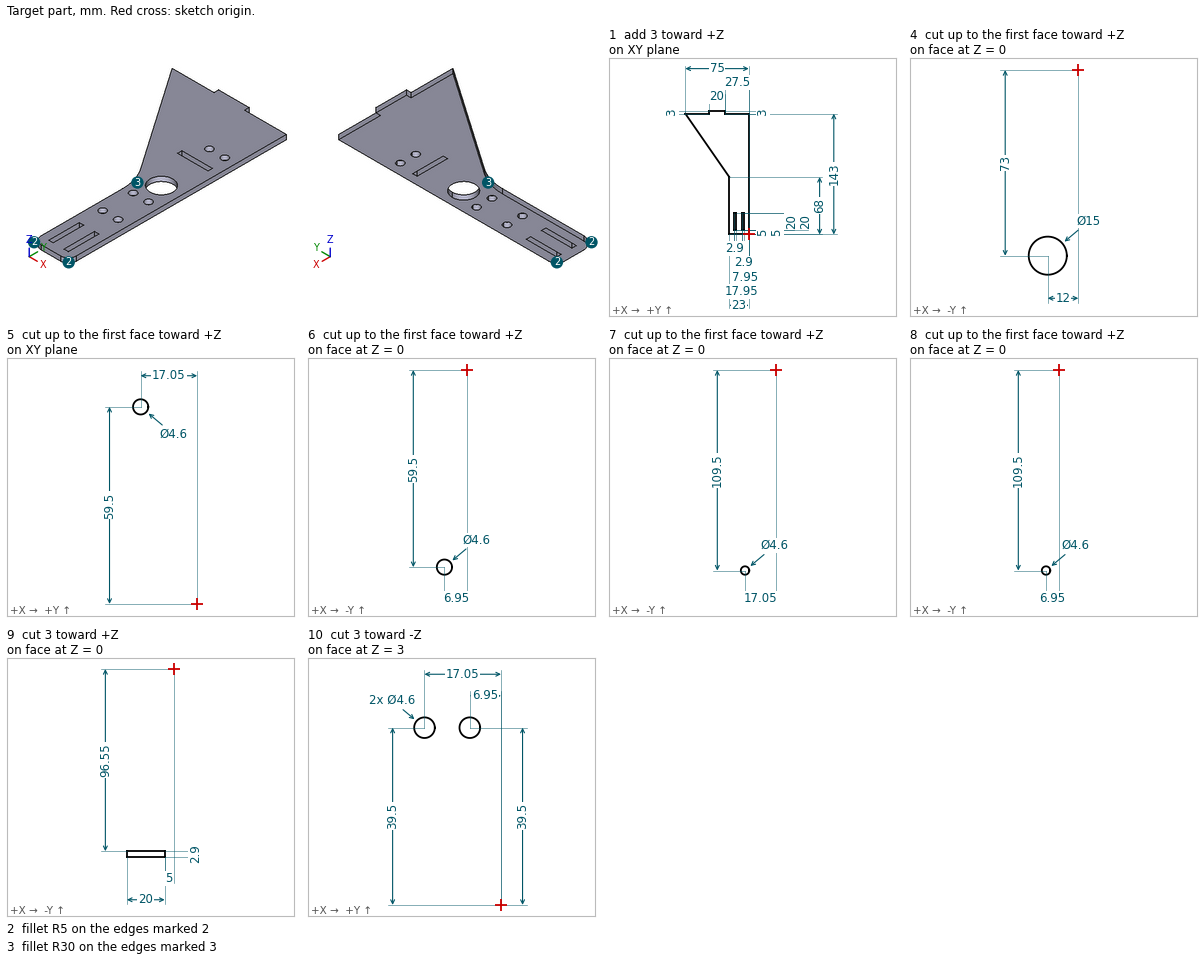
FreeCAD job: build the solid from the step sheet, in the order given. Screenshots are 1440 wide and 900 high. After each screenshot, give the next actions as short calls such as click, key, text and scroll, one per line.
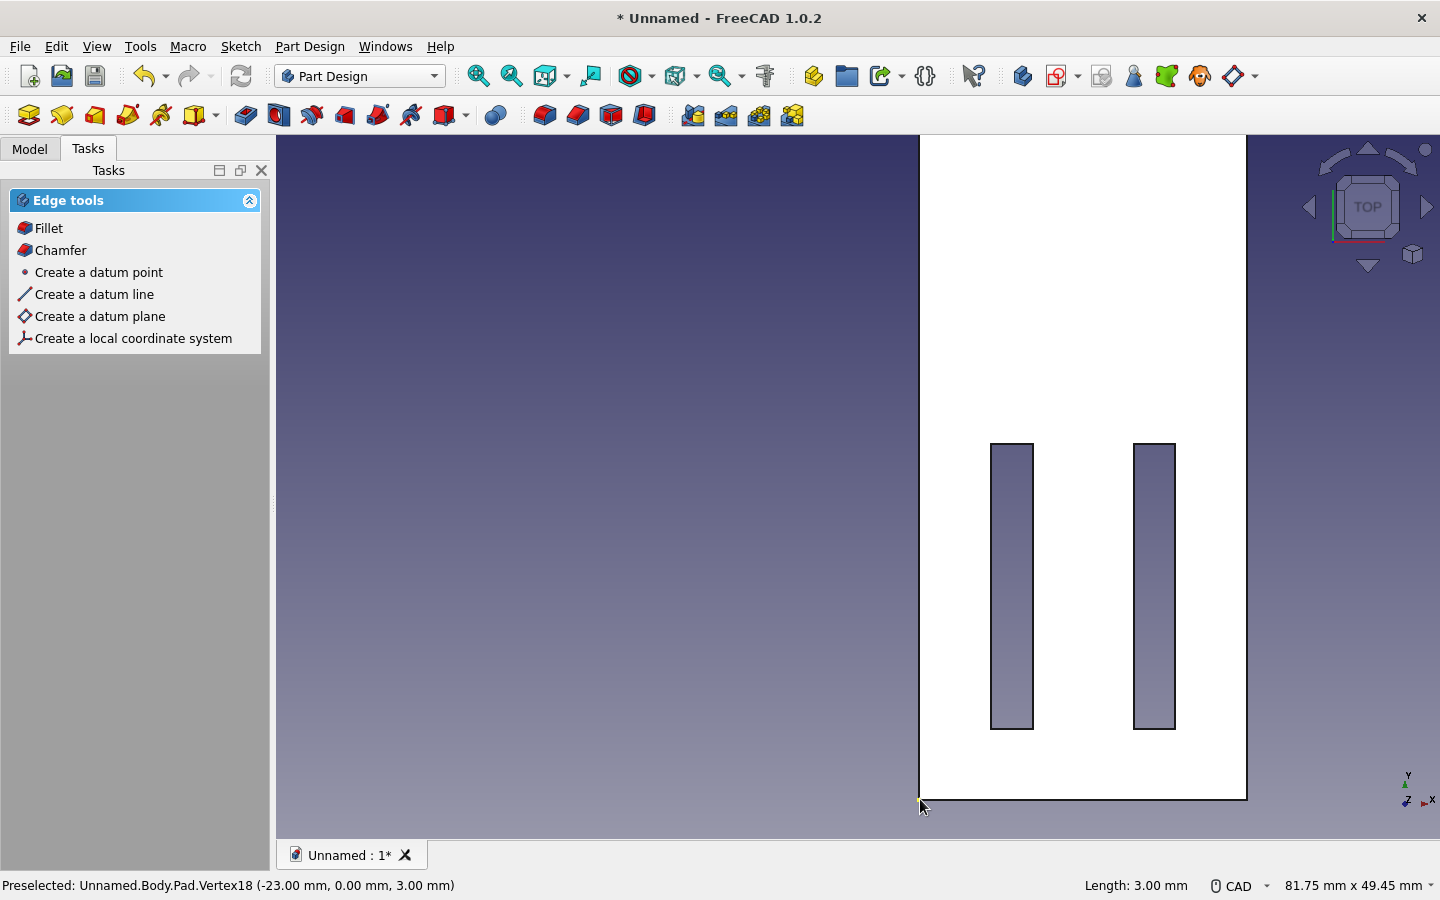
key(v)
key(f)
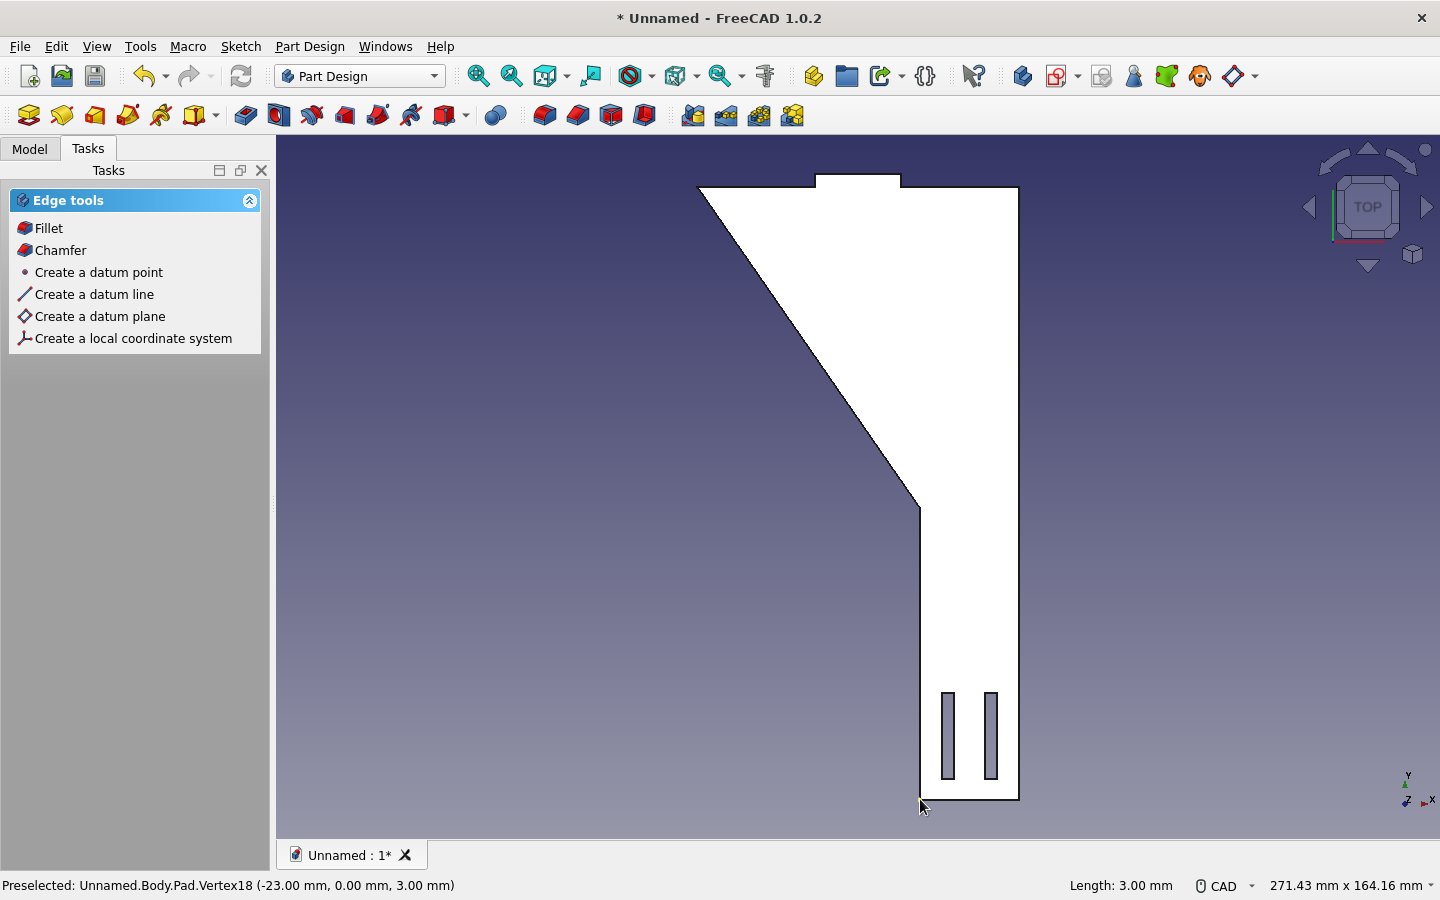
key(1)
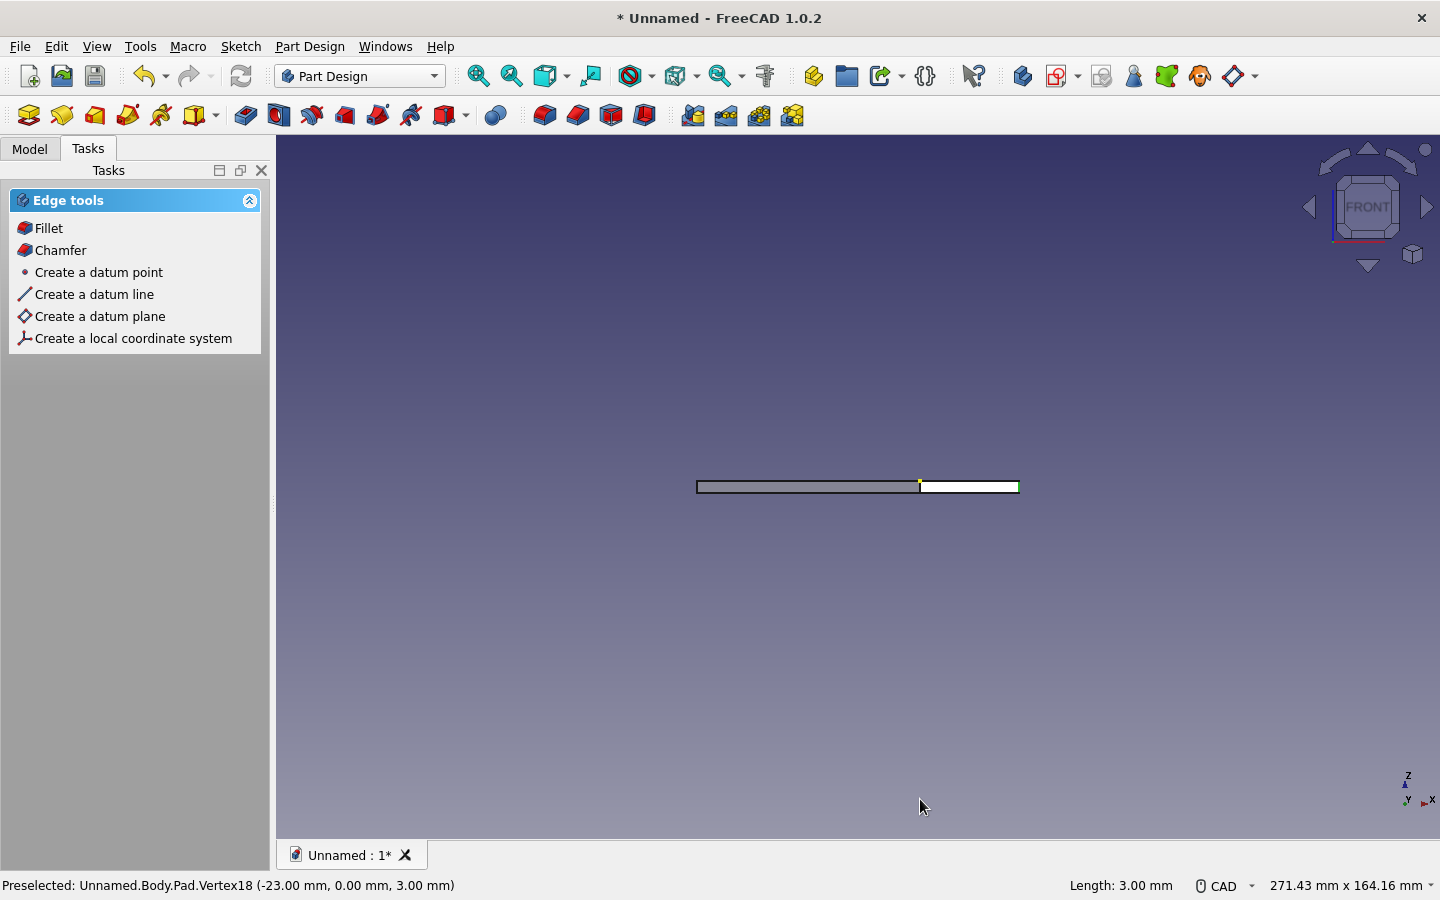
key(v)
key(f)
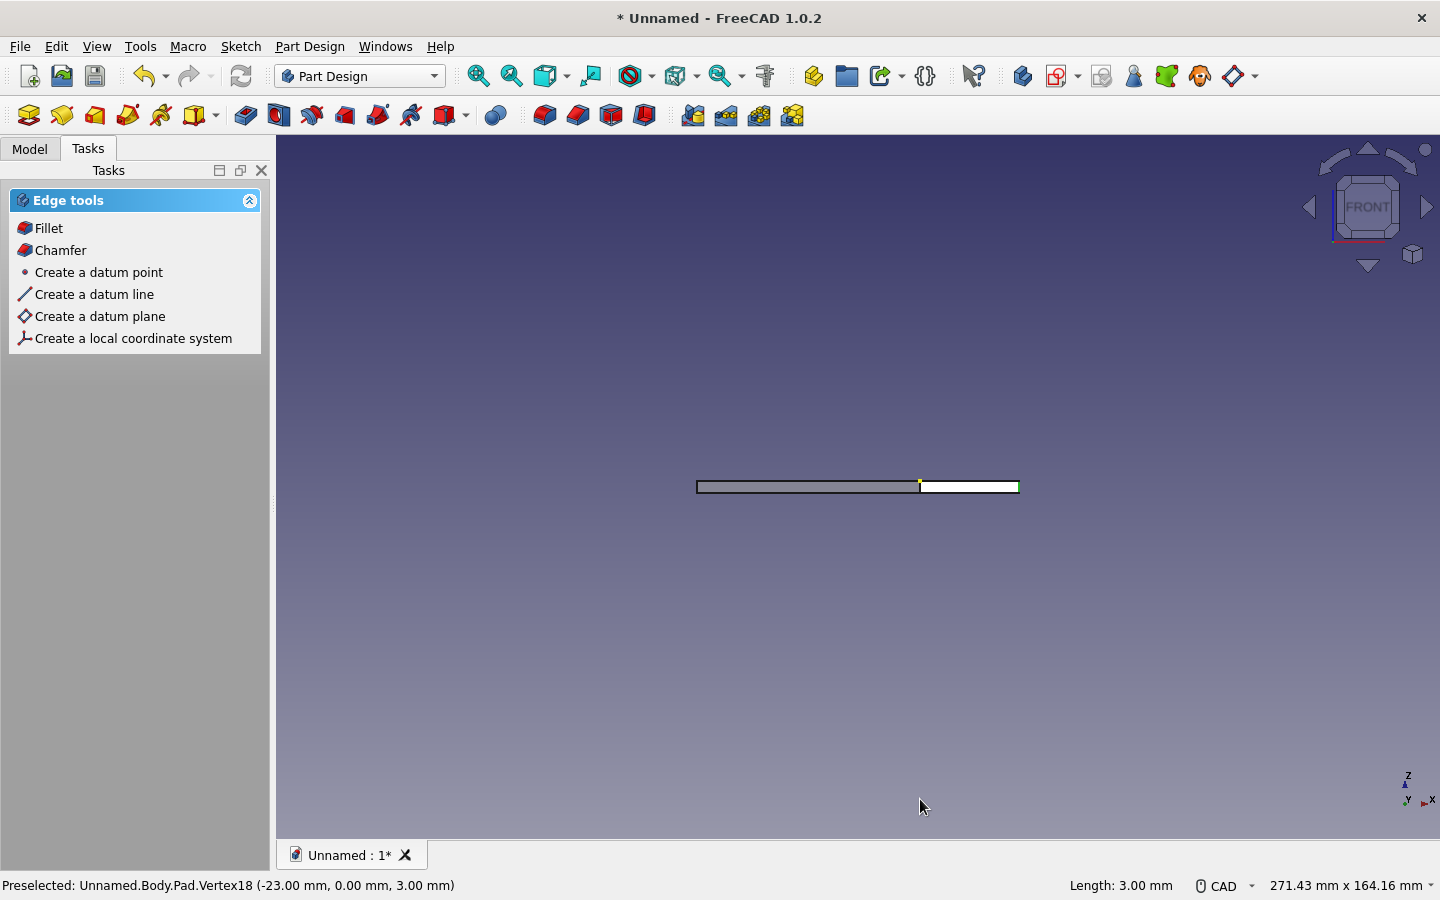
click(920, 486, ctrl)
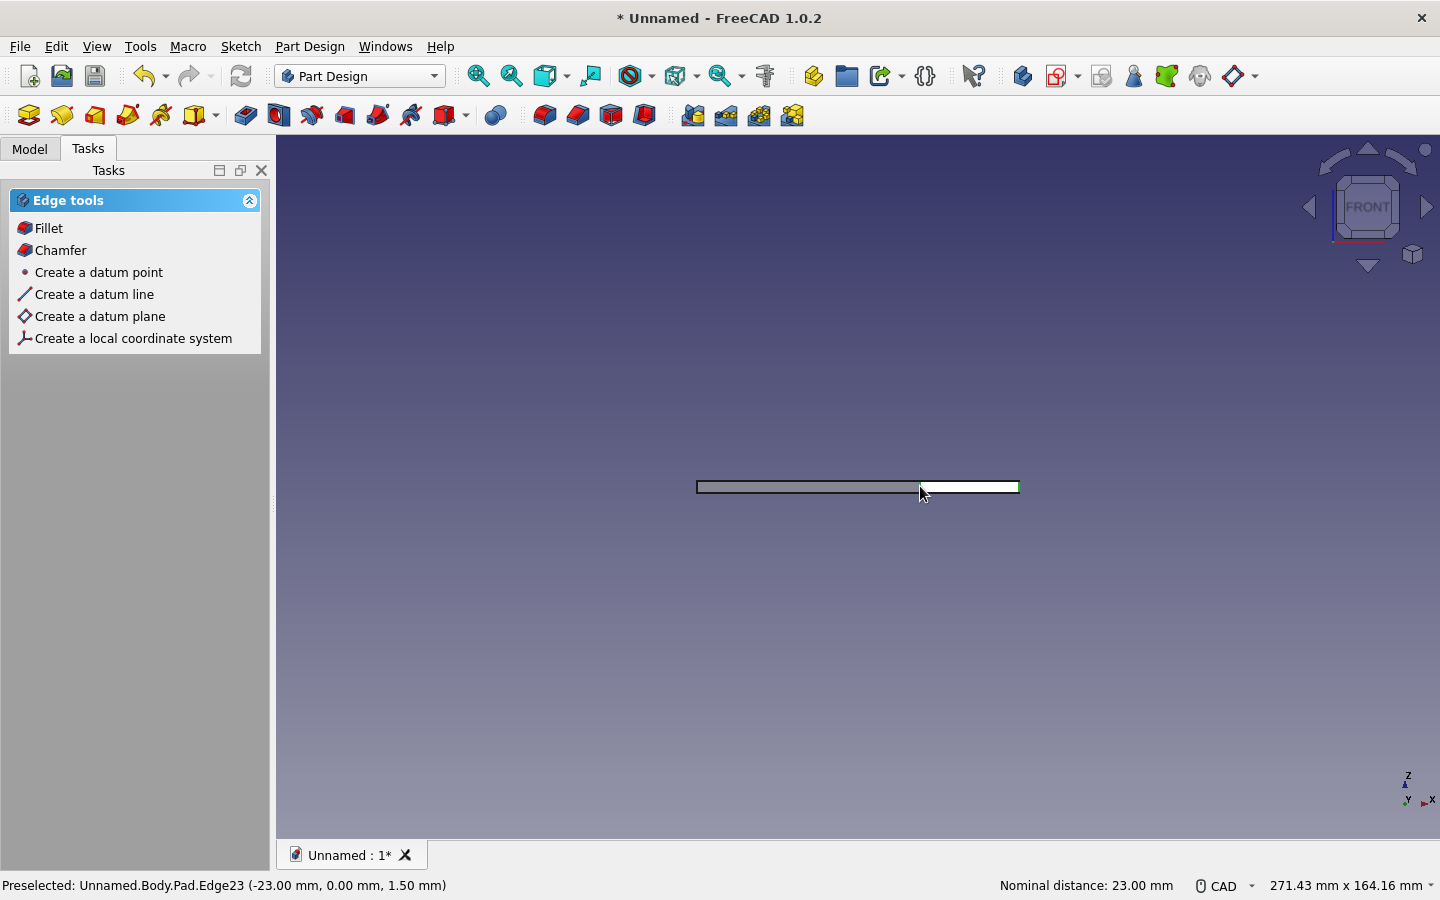
click(545, 116)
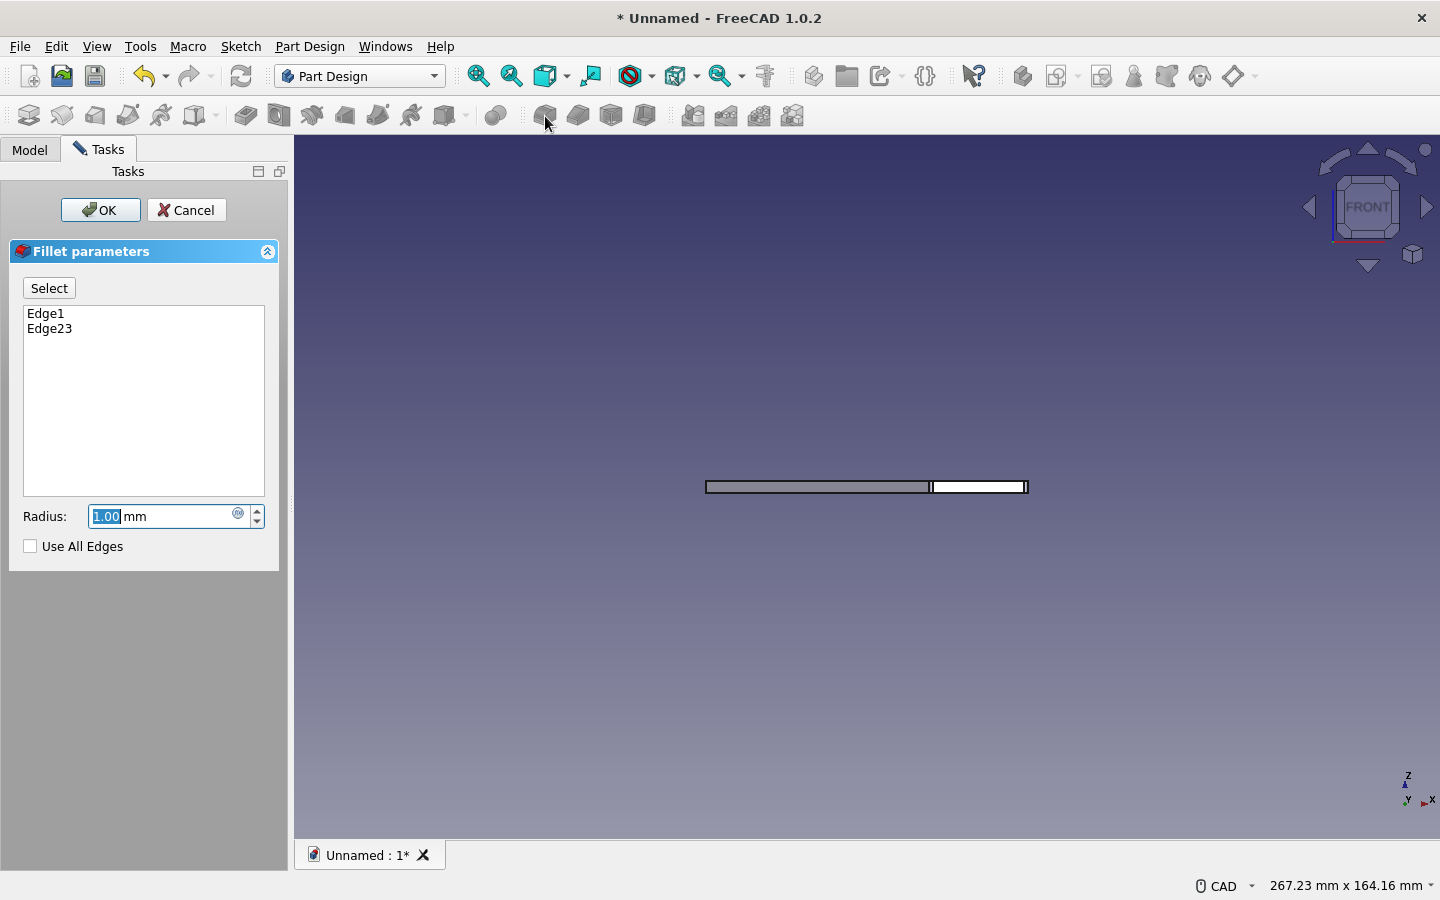
text(5)
key(Tab)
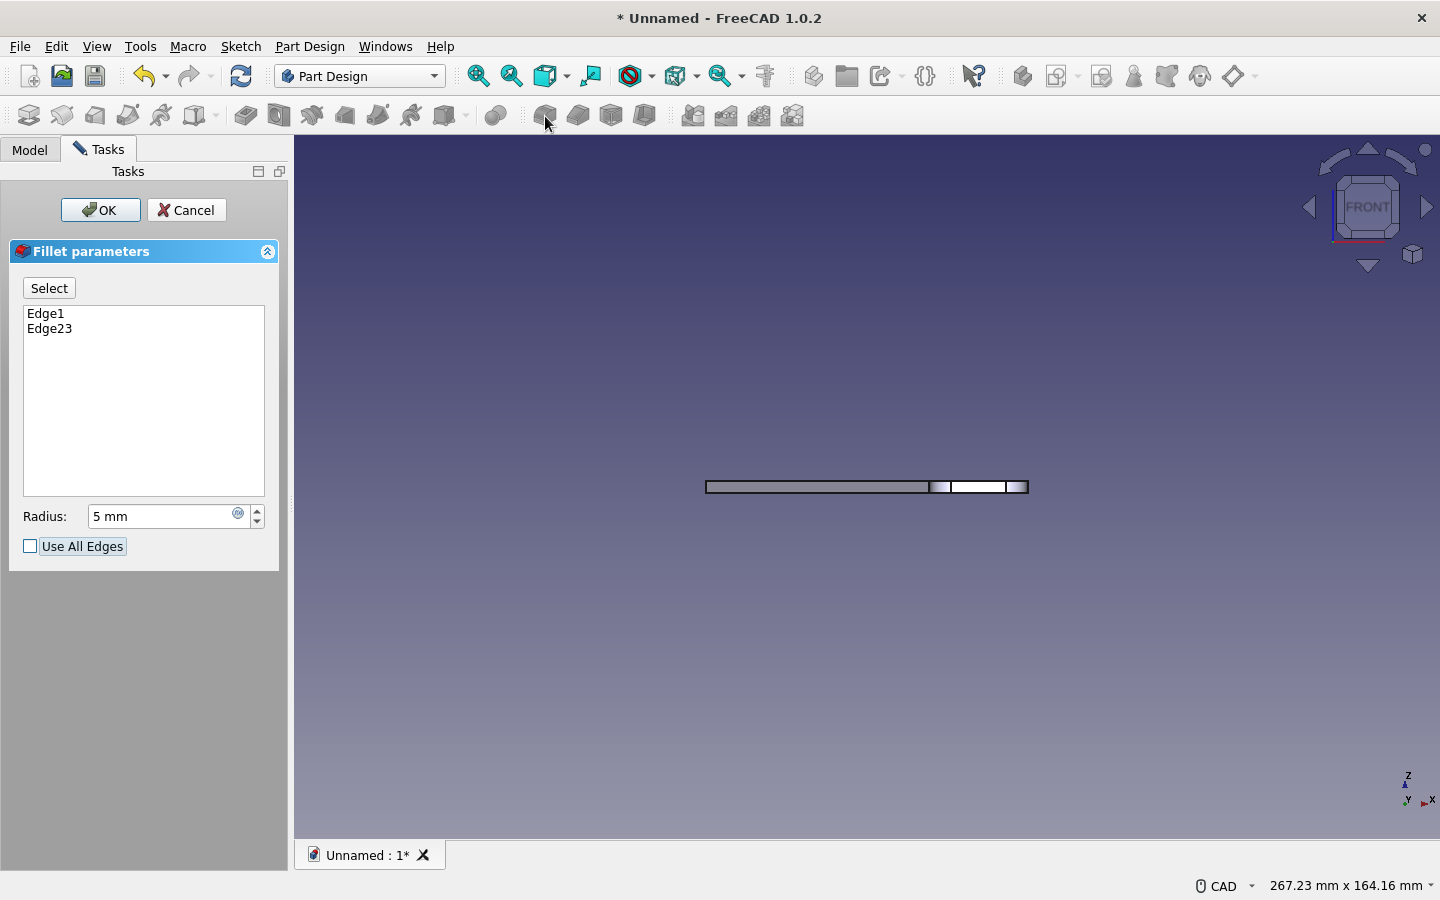
click(101, 210)